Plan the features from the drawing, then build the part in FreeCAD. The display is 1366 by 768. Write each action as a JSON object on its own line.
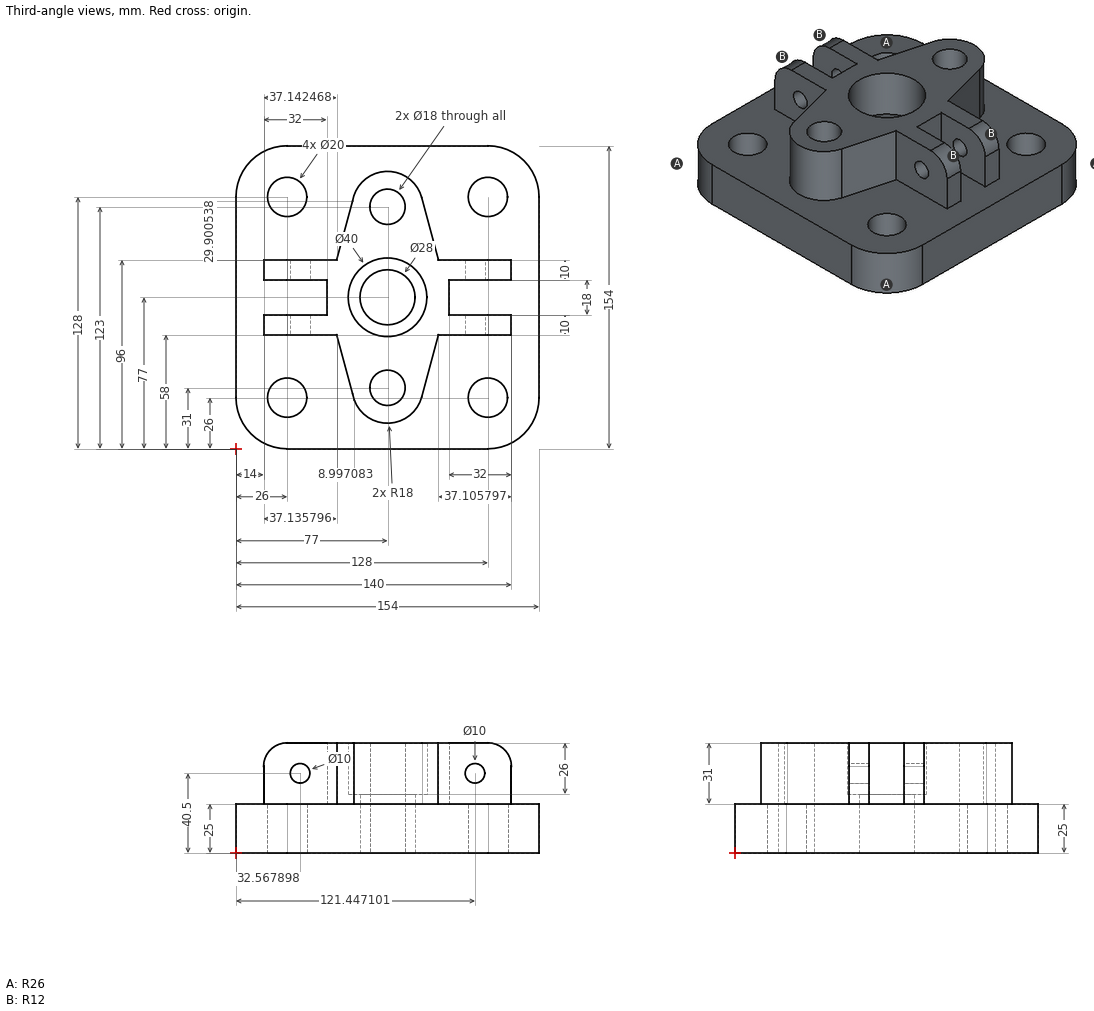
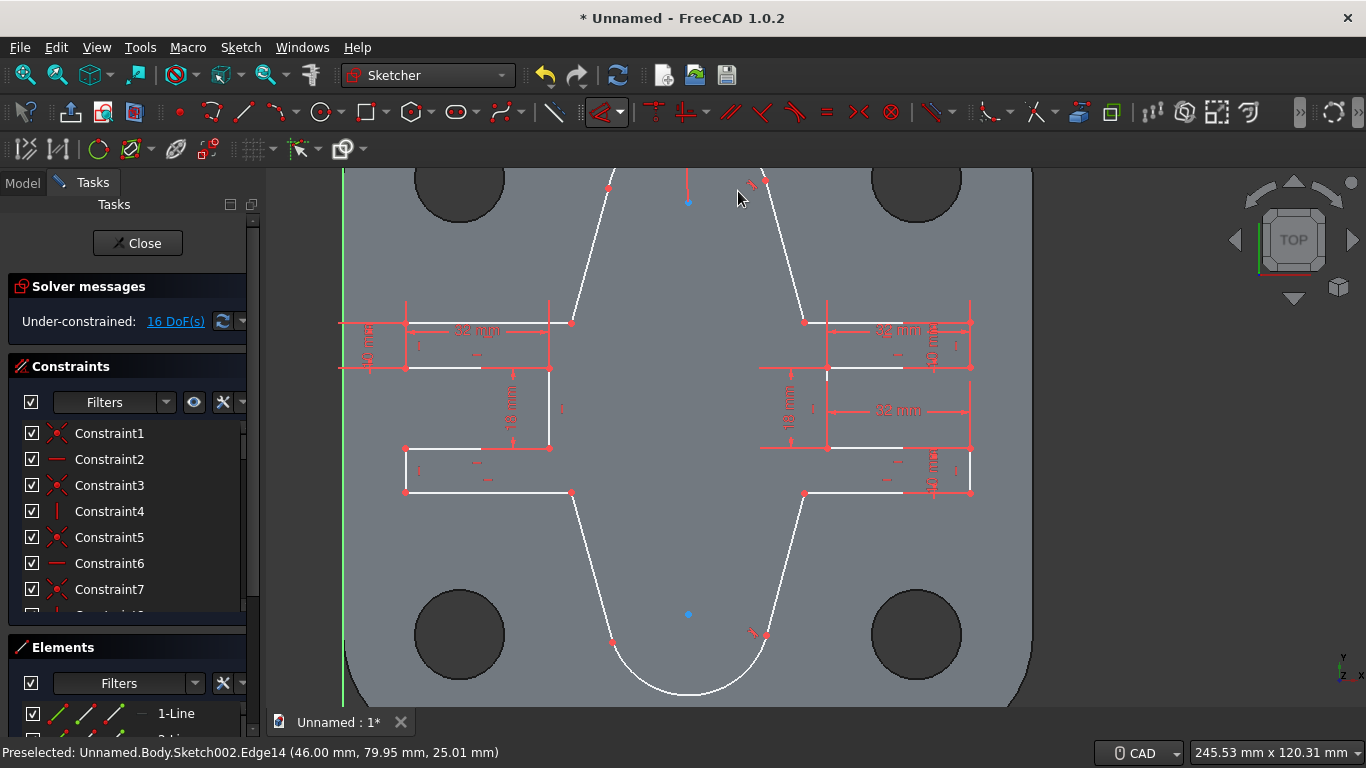
{"action": "left_click", "coordinate": [506, 449]}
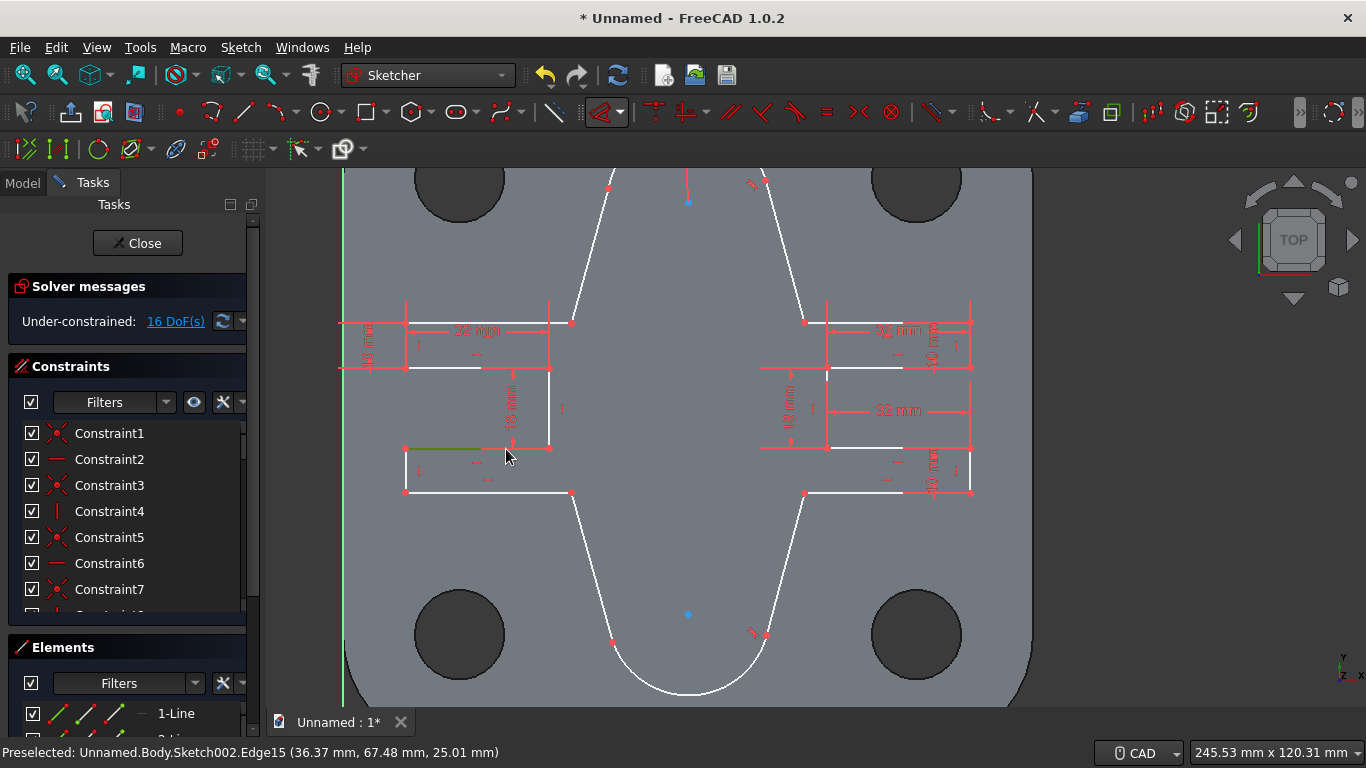
{"action": "key", "text": "l"}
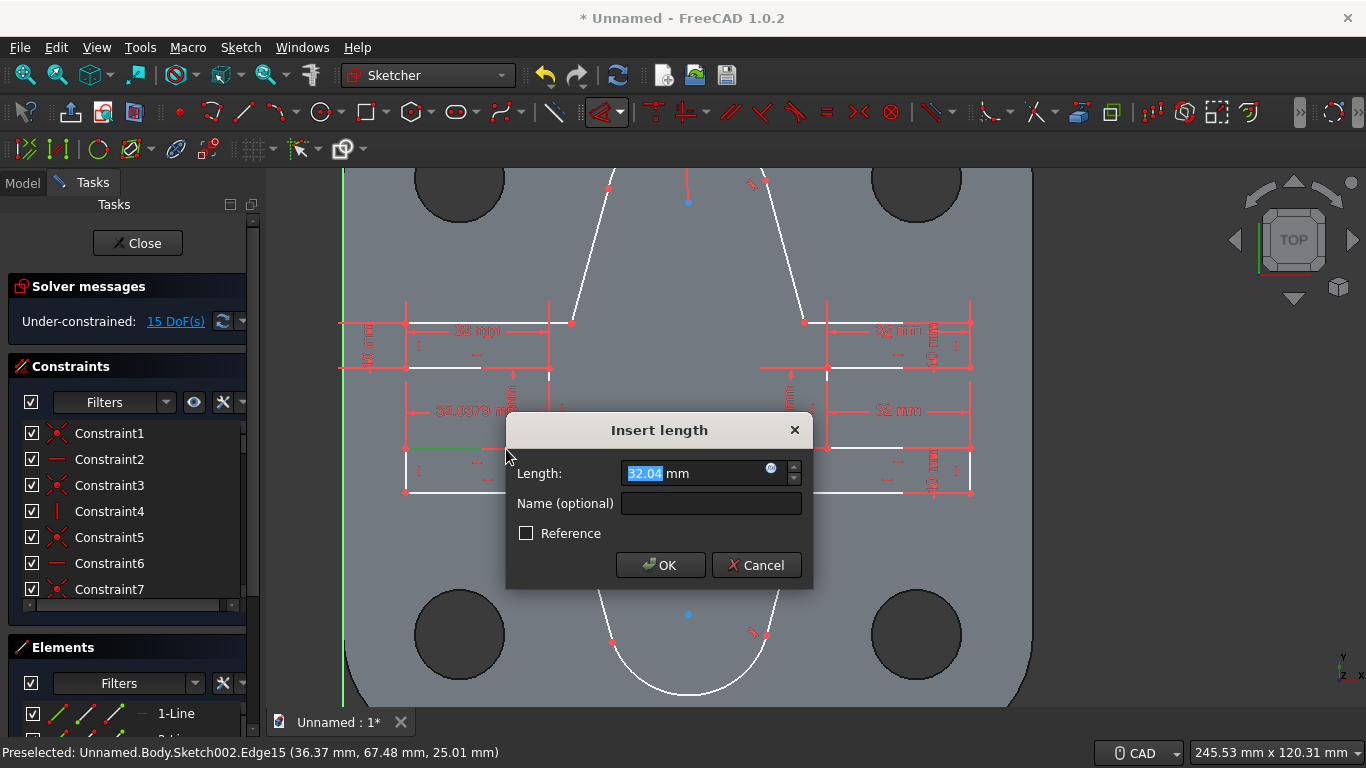
{"action": "type", "text": "32"}
{"action": "key", "text": "Return"}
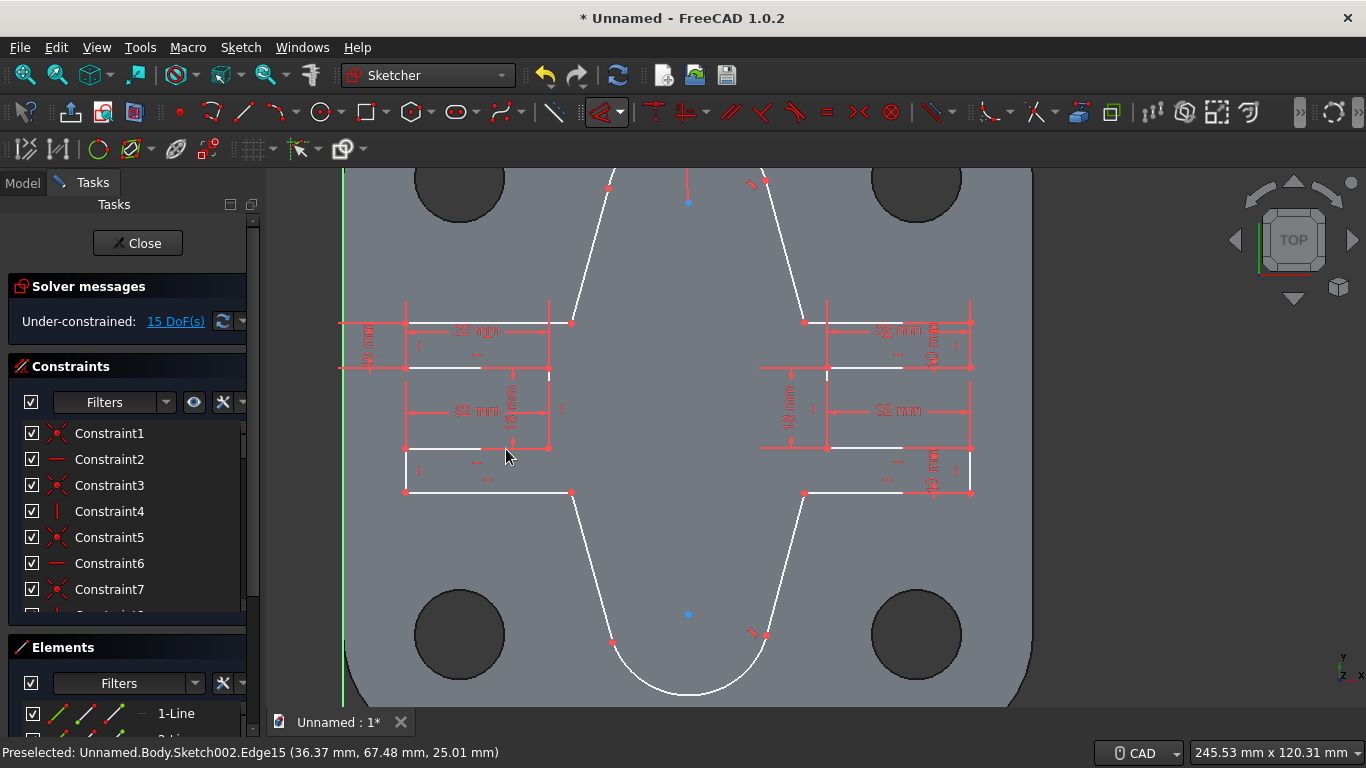
{"action": "left_click", "coordinate": [406, 462]}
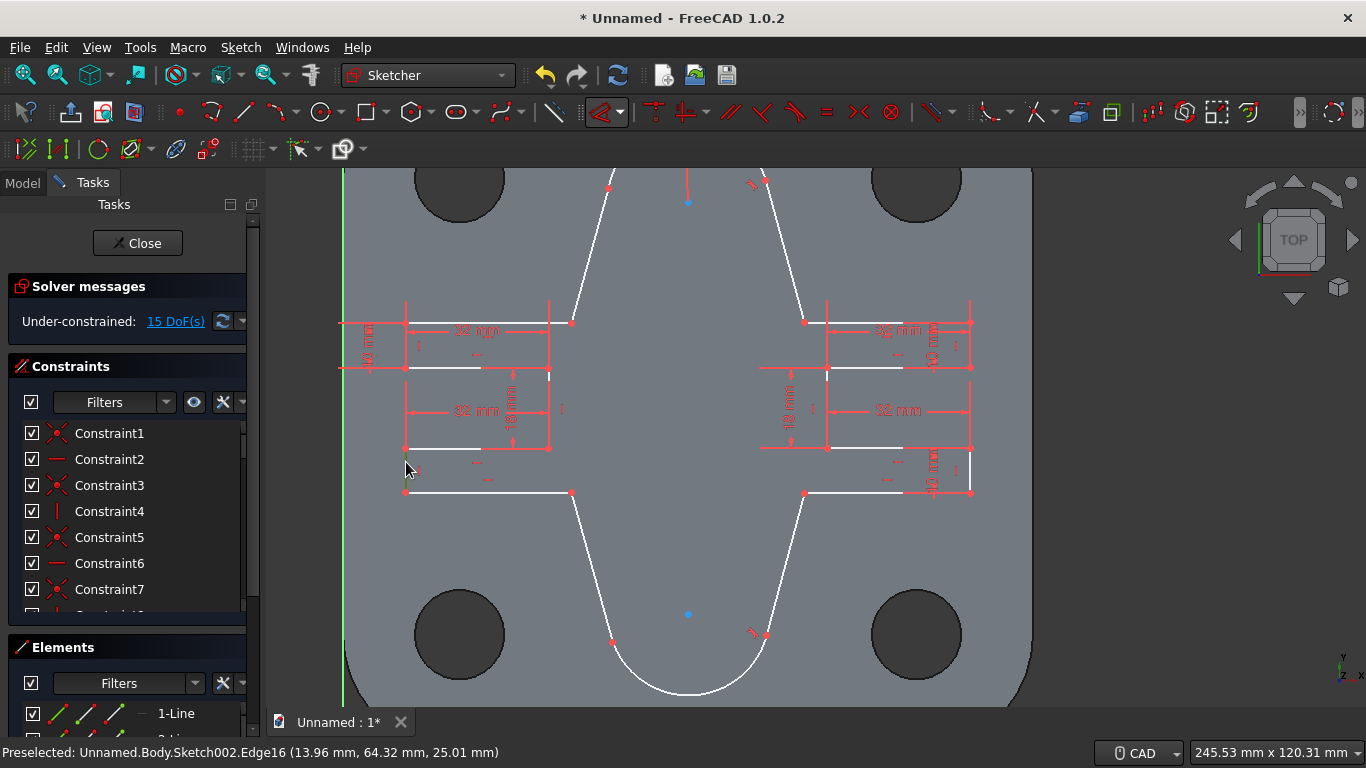
{"action": "left_click", "coordinate": [622, 112]}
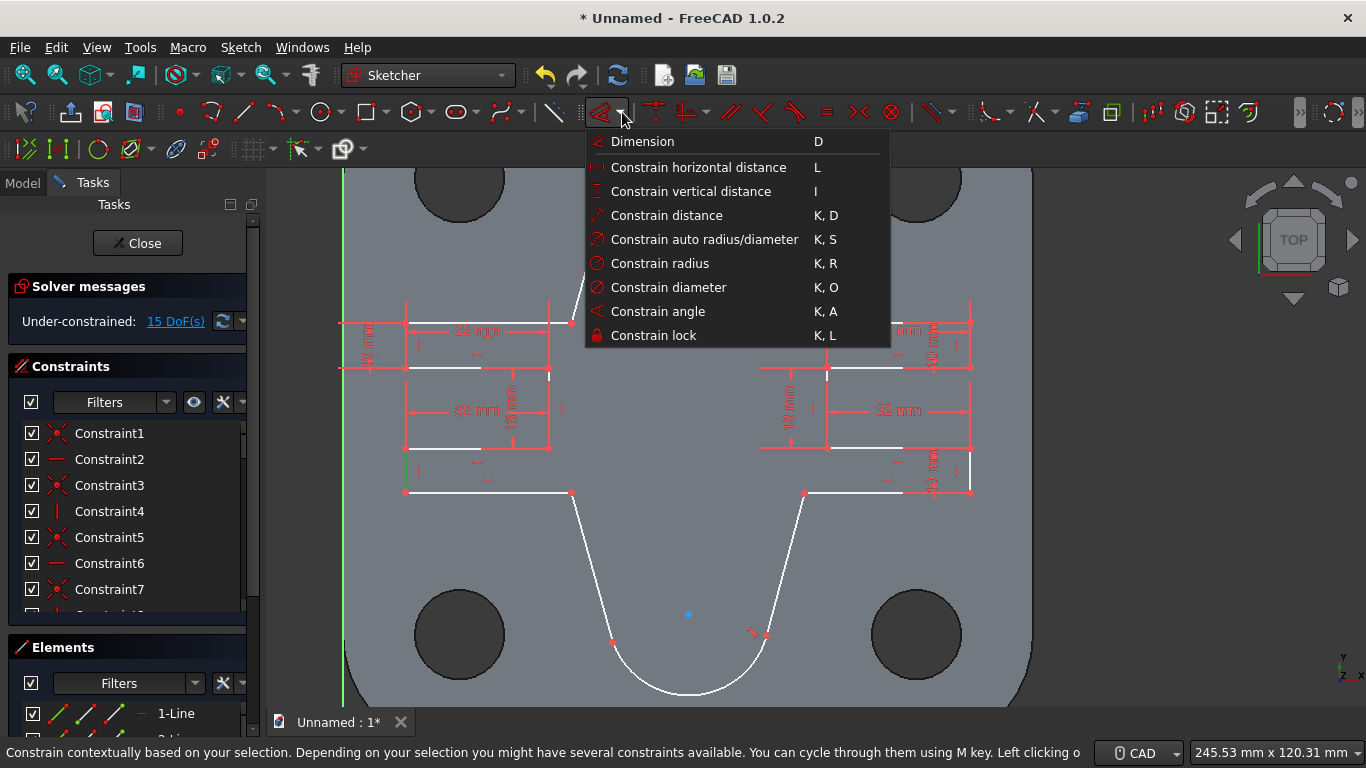
{"action": "left_click", "coordinate": [738, 191]}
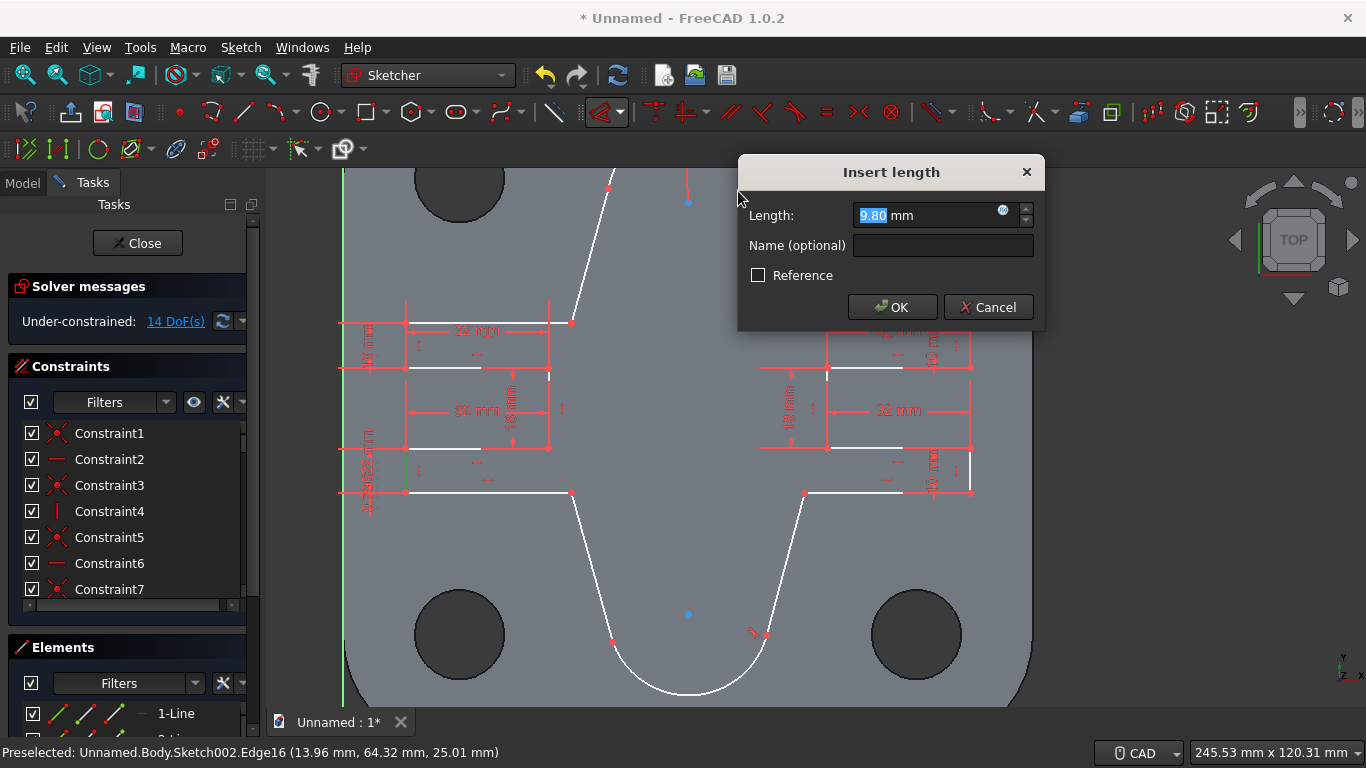
{"action": "type", "text": "10"}
{"action": "key", "text": "Return"}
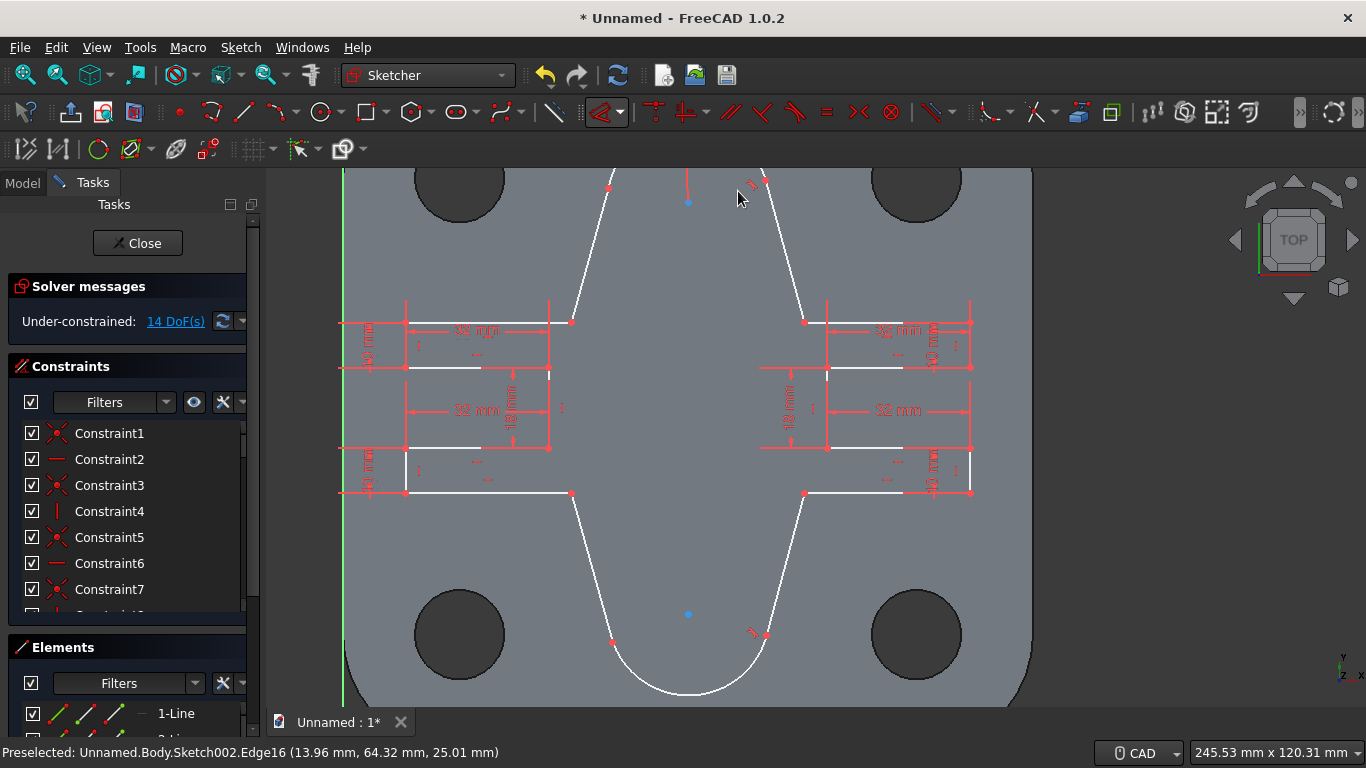
{"action": "left_click", "coordinate": [805, 493]}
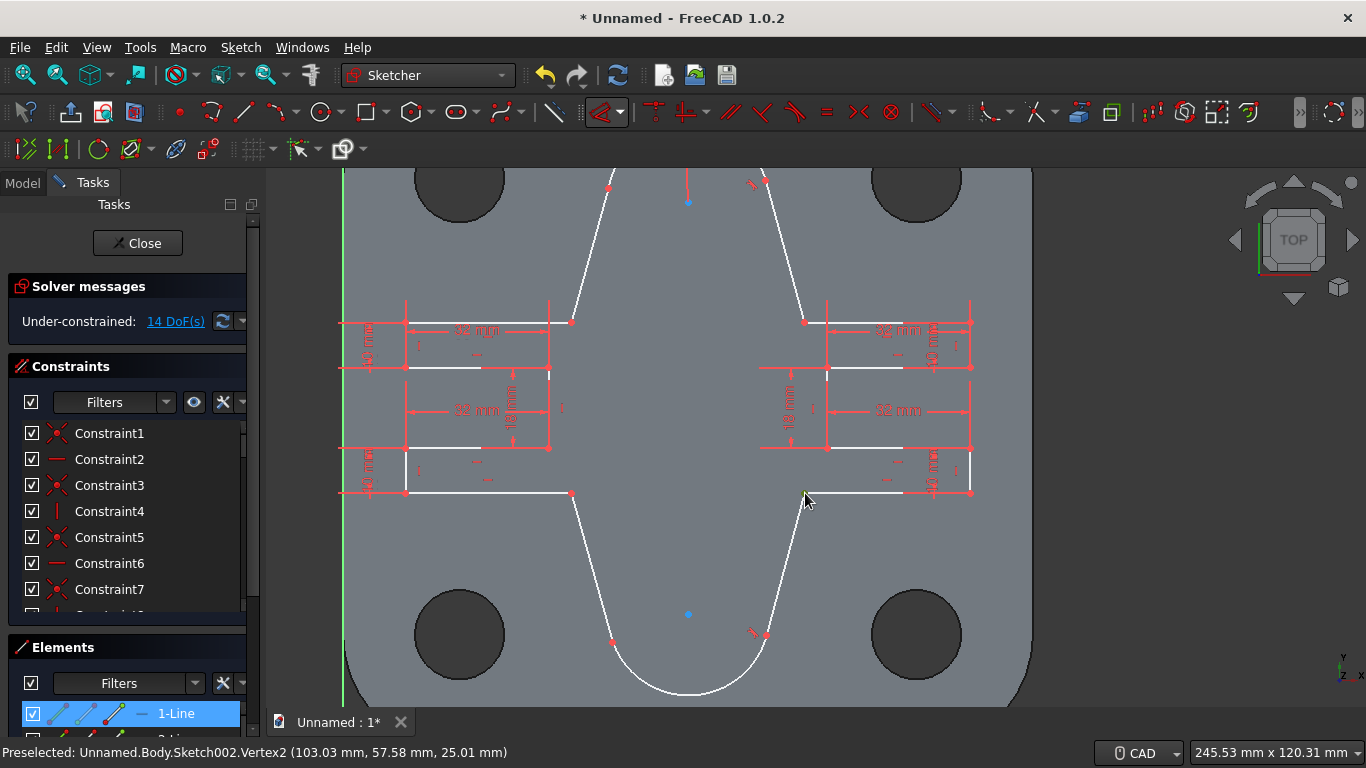
{"action": "key", "text": "i"}